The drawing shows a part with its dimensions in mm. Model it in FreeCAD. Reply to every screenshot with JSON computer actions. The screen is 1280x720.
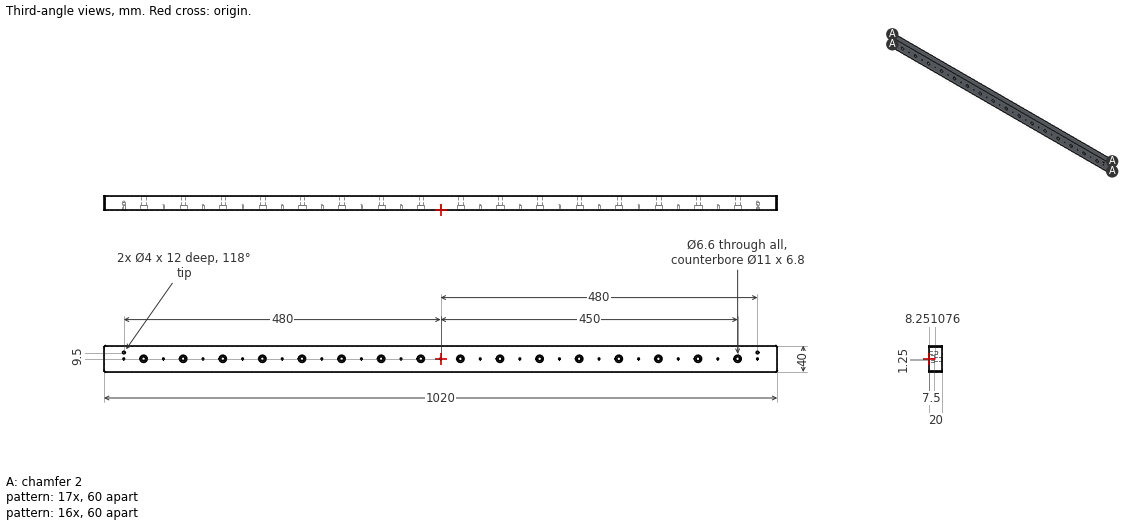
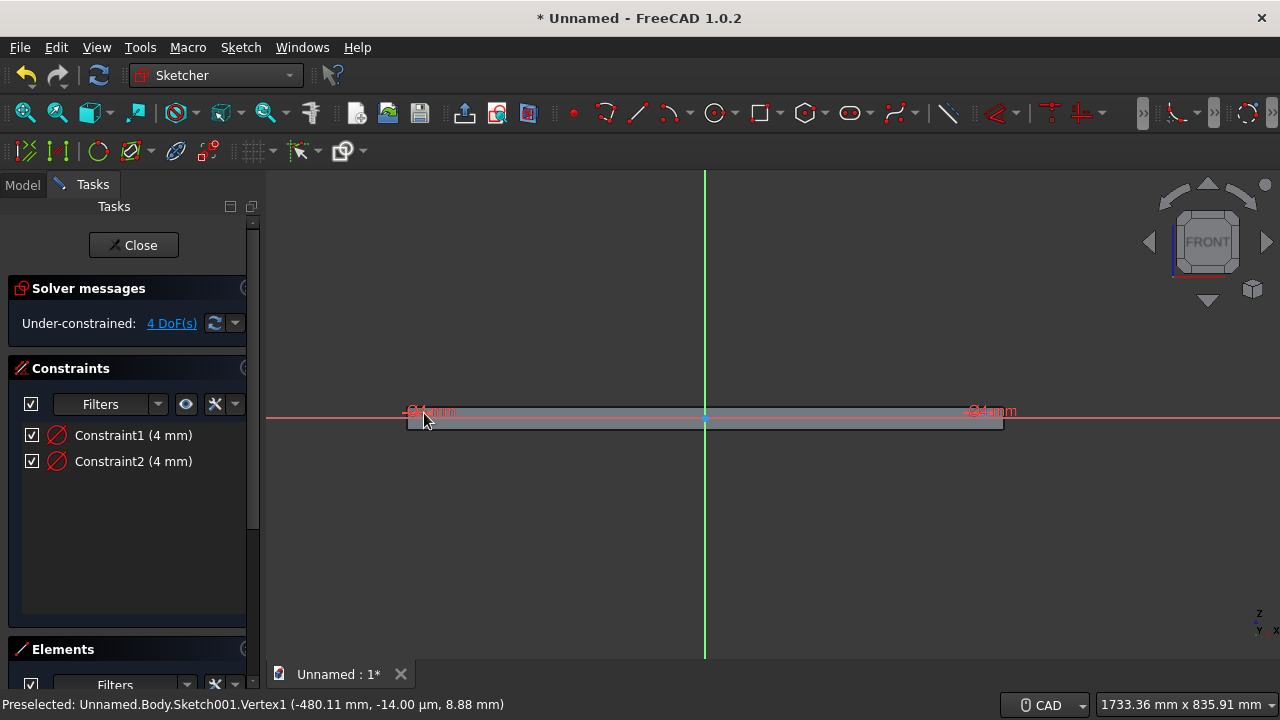
{"action": "left_click", "coordinate": [986, 413]}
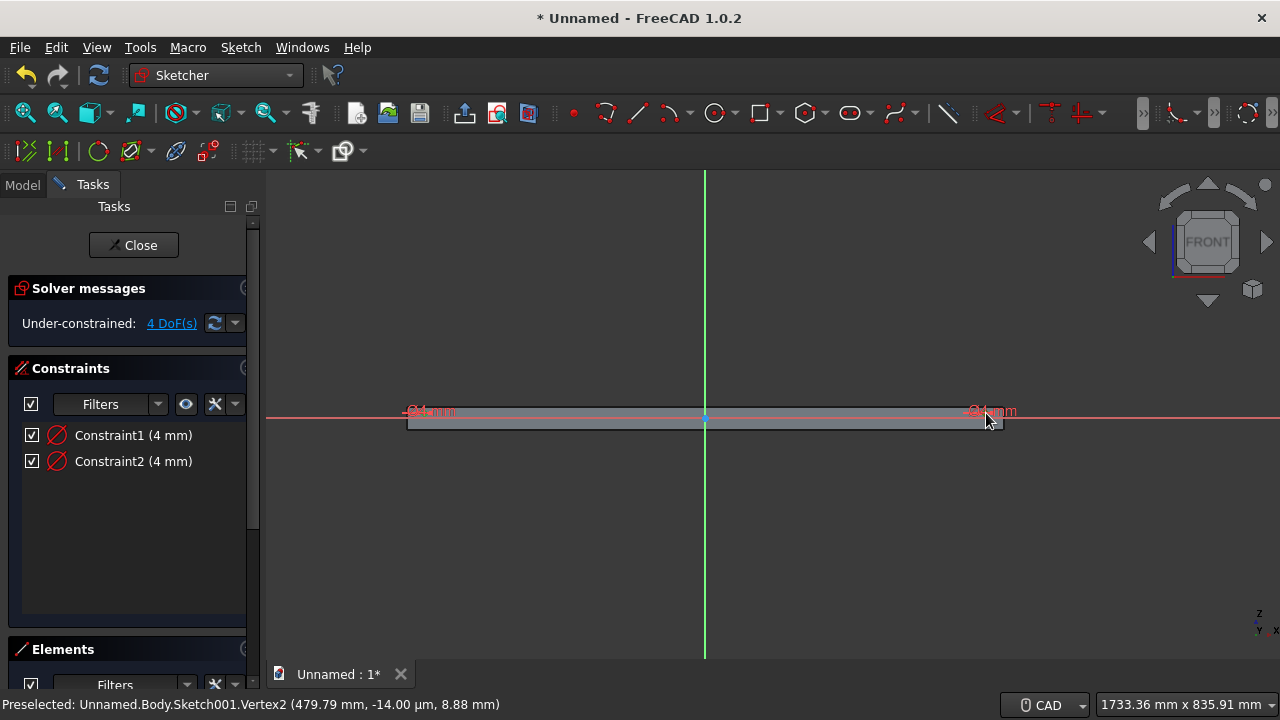
{"action": "key", "text": "h"}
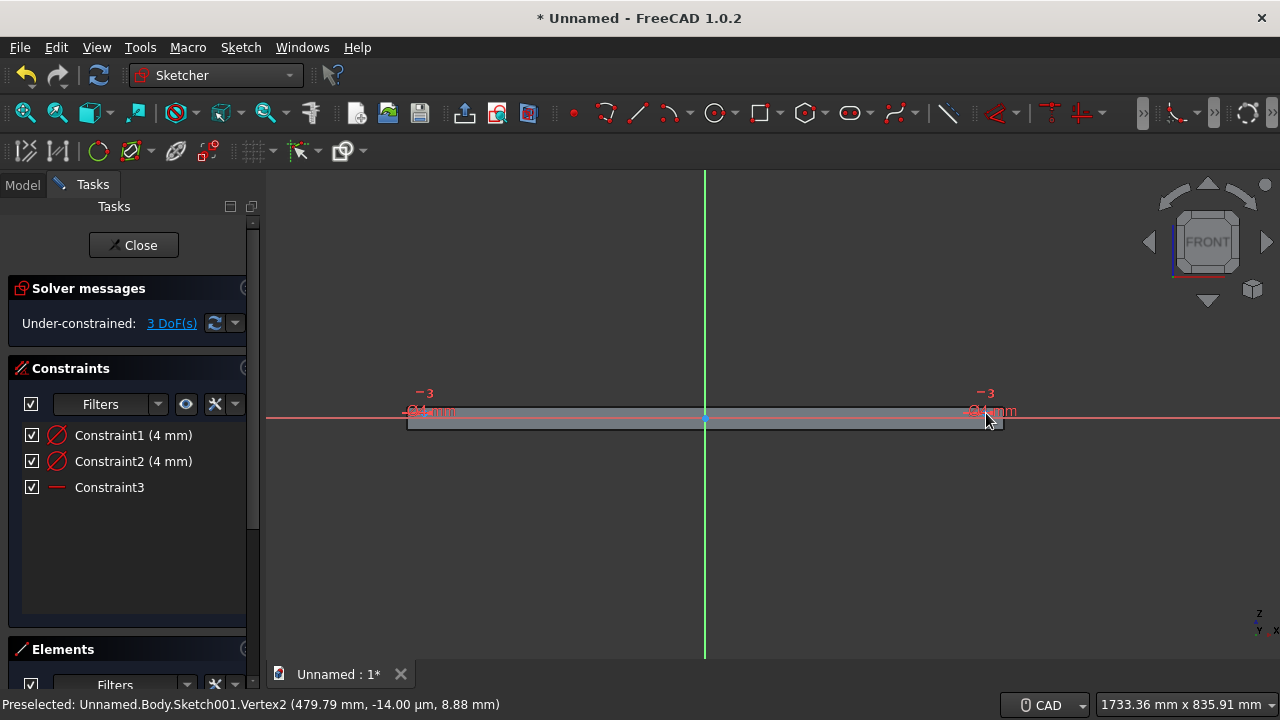
{"action": "key", "text": "d"}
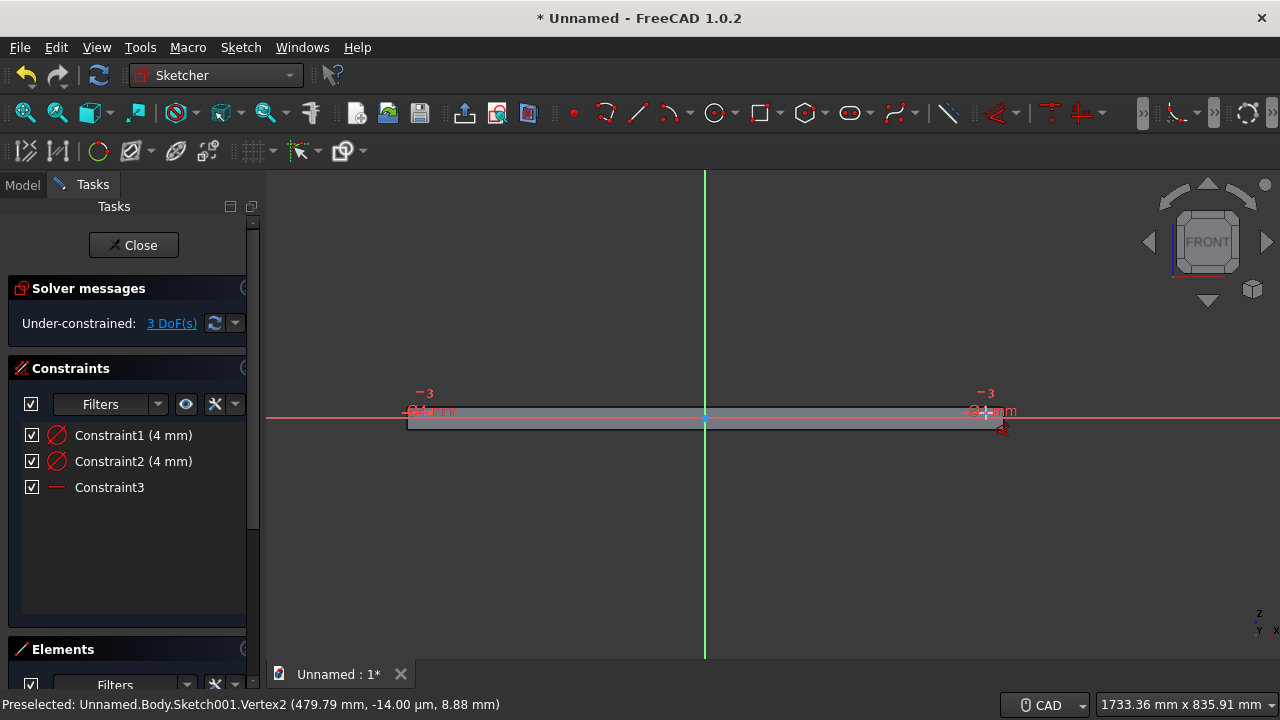
{"action": "left_click", "coordinate": [424, 413]}
{"action": "left_click", "coordinate": [565, 452]}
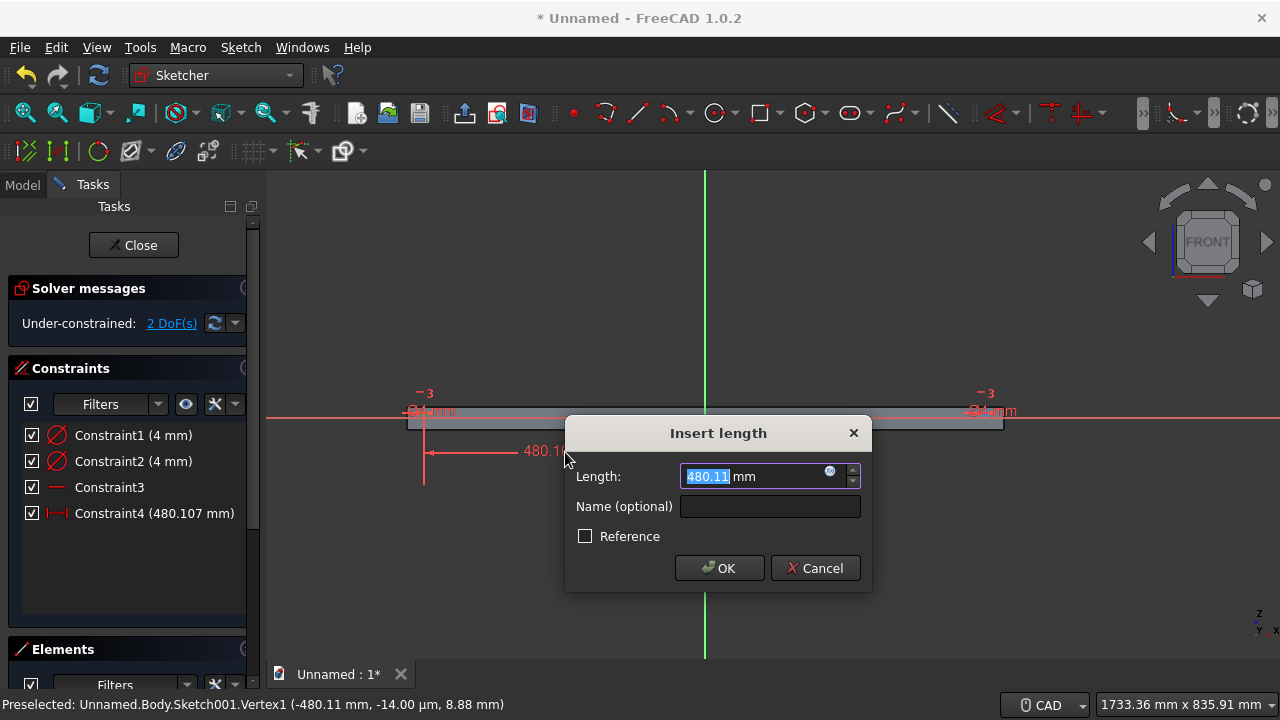
{"action": "type", "text": "480"}
{"action": "key", "text": "Return"}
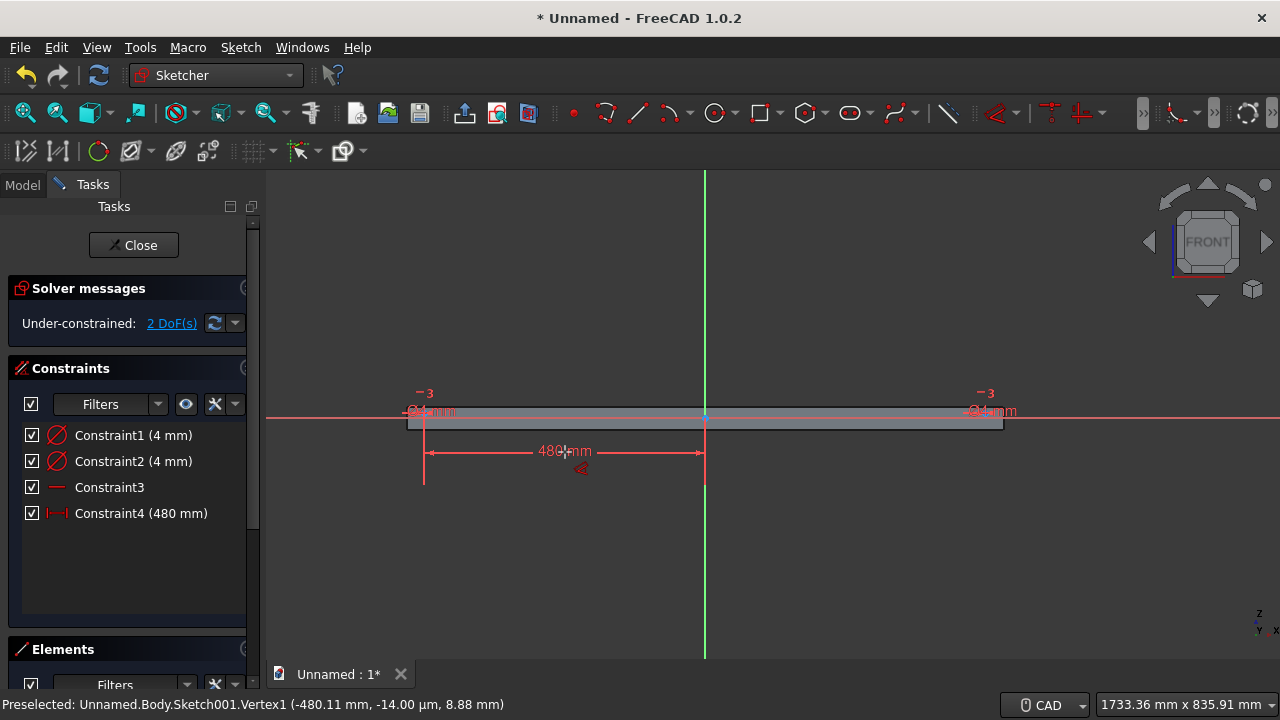
{"action": "scroll", "coordinate": [424, 413], "scroll_direction": "up", "scroll_amount": 10}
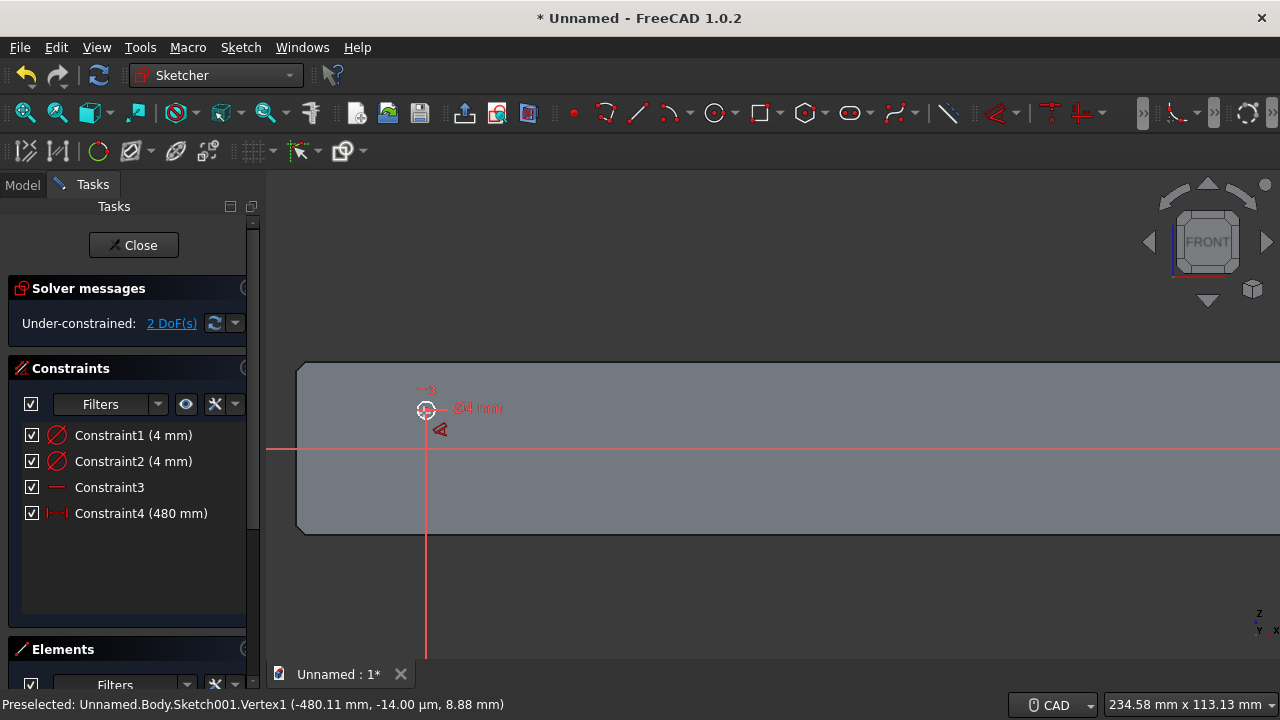
{"action": "left_click", "coordinate": [426, 410]}
{"action": "left_click", "coordinate": [392, 429]}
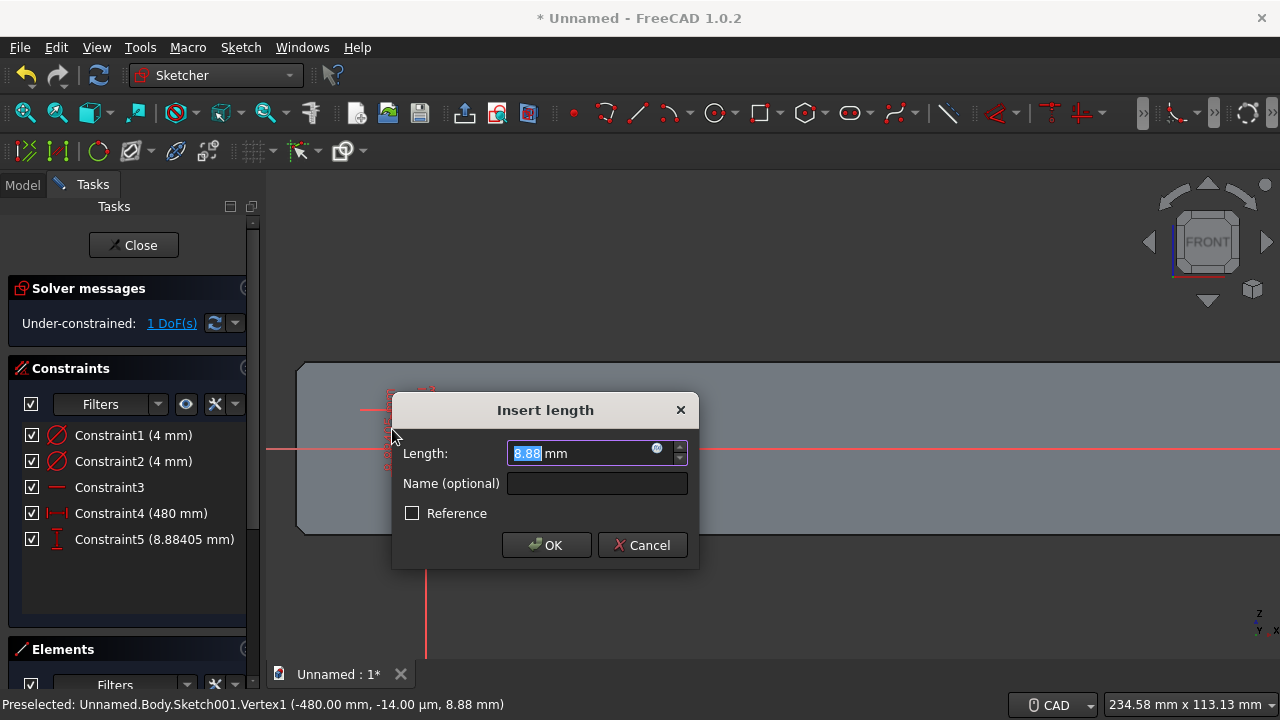
{"action": "type", "text": "9.5"}
{"action": "key", "text": "Return"}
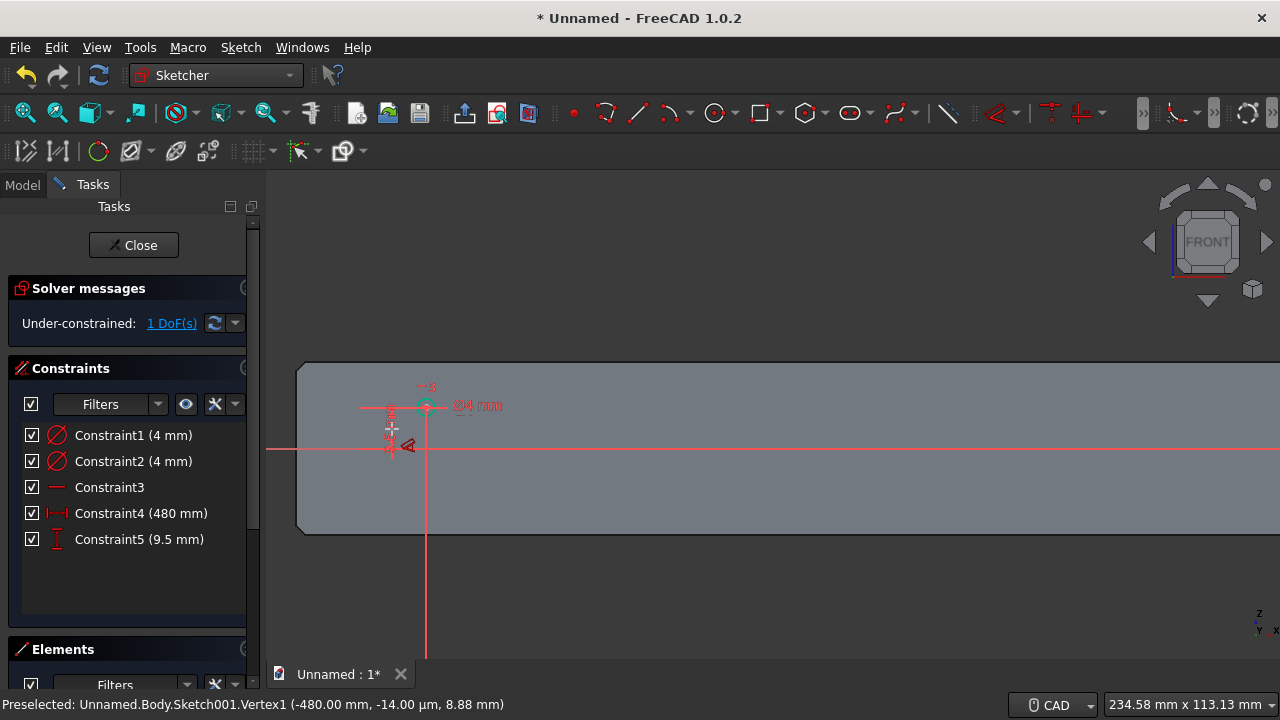
{"action": "scroll", "coordinate": [423, 413], "scroll_direction": "down", "scroll_amount": 10}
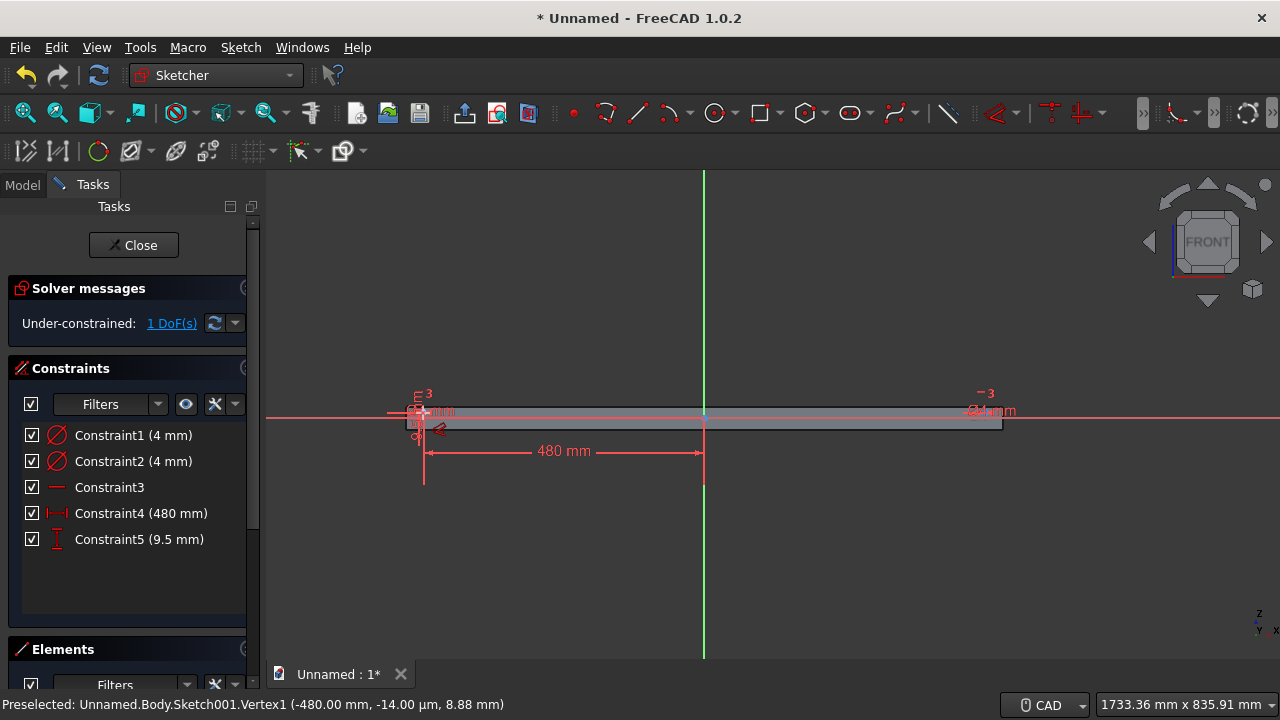
{"action": "left_click", "coordinate": [985, 413]}
{"action": "left_click", "coordinate": [845, 452]}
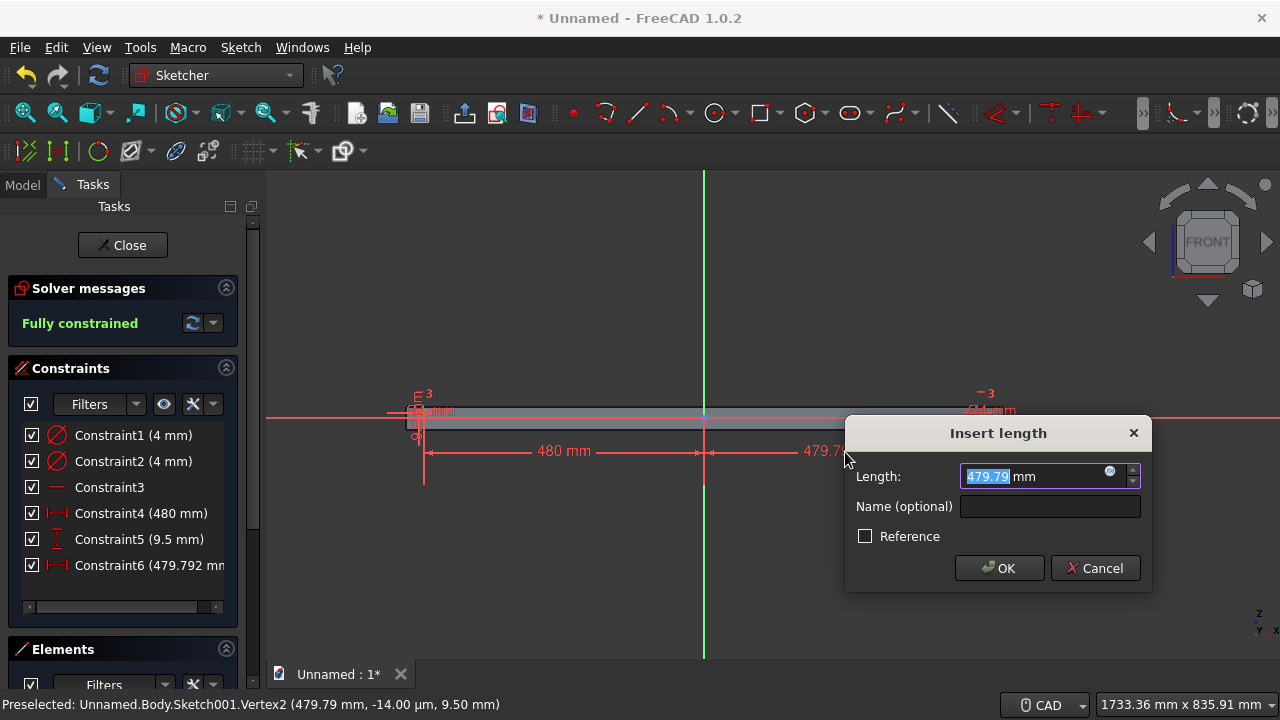
{"action": "type", "text": "480"}
{"action": "key", "text": "Return"}
{"action": "key", "text": "Escape"}